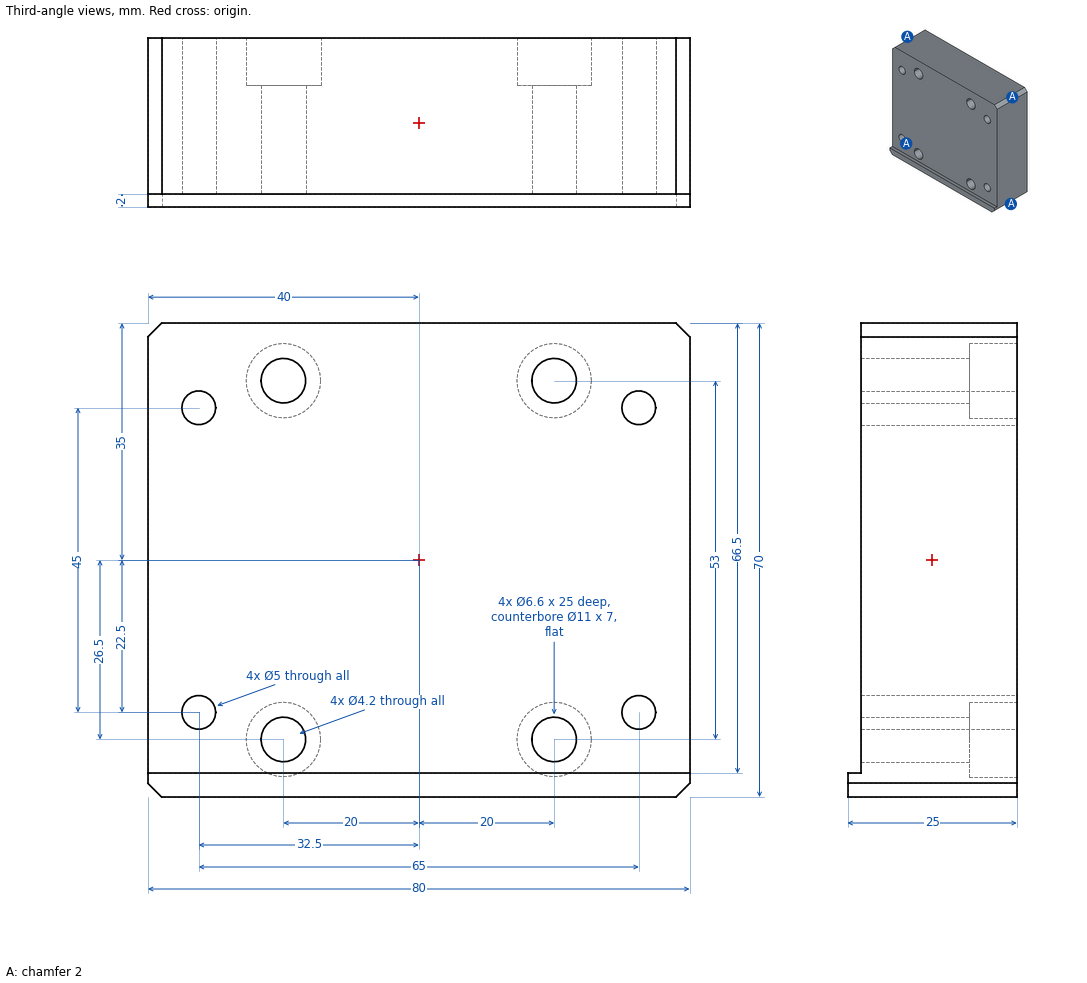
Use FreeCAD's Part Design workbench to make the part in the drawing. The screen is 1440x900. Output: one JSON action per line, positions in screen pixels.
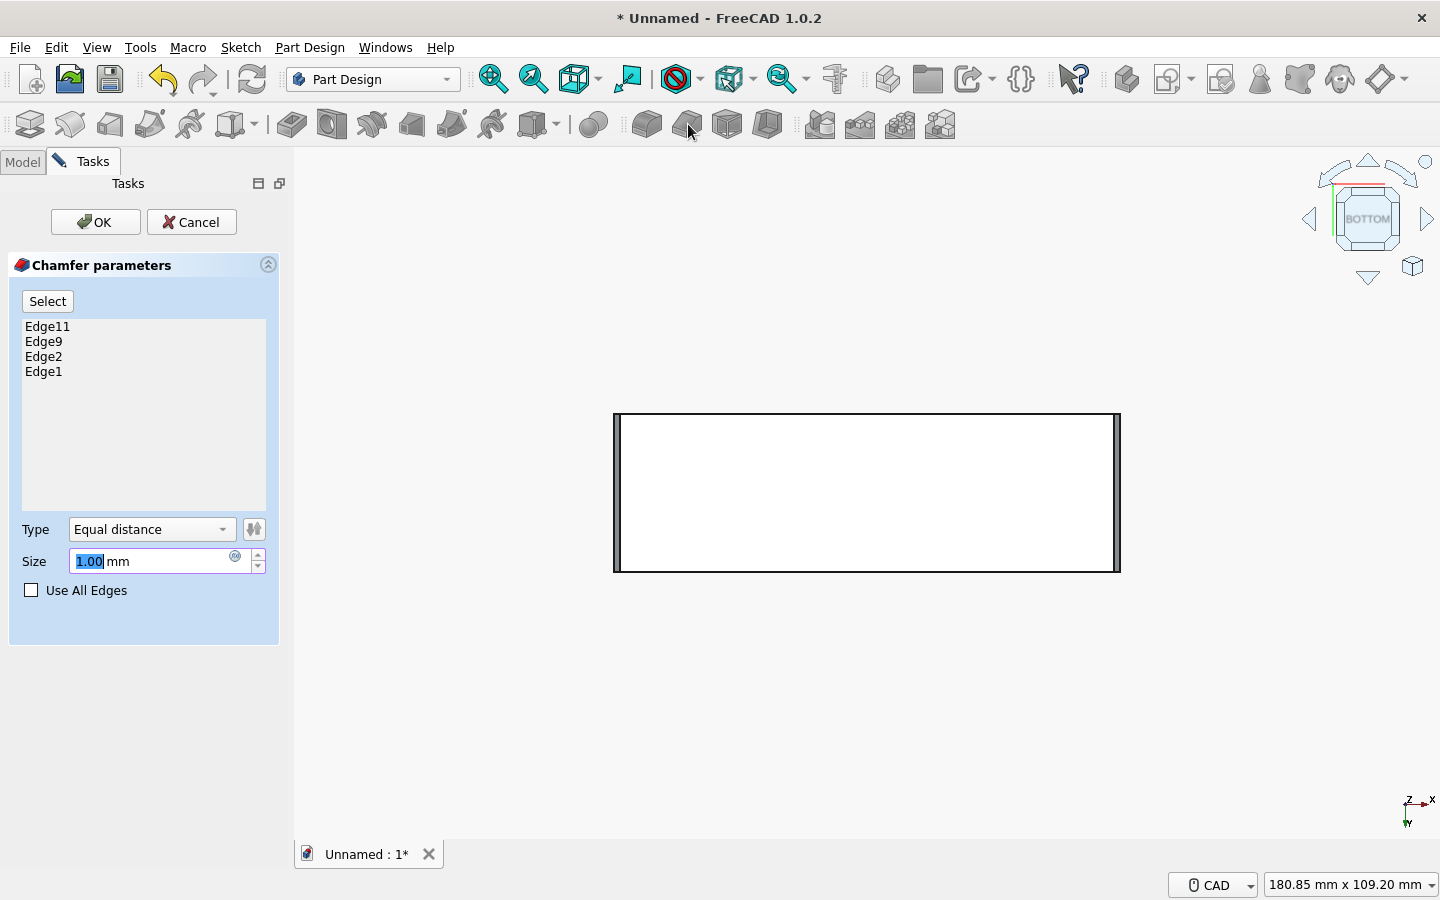
{"action": "type", "text": "2"}
{"action": "key", "text": "Tab"}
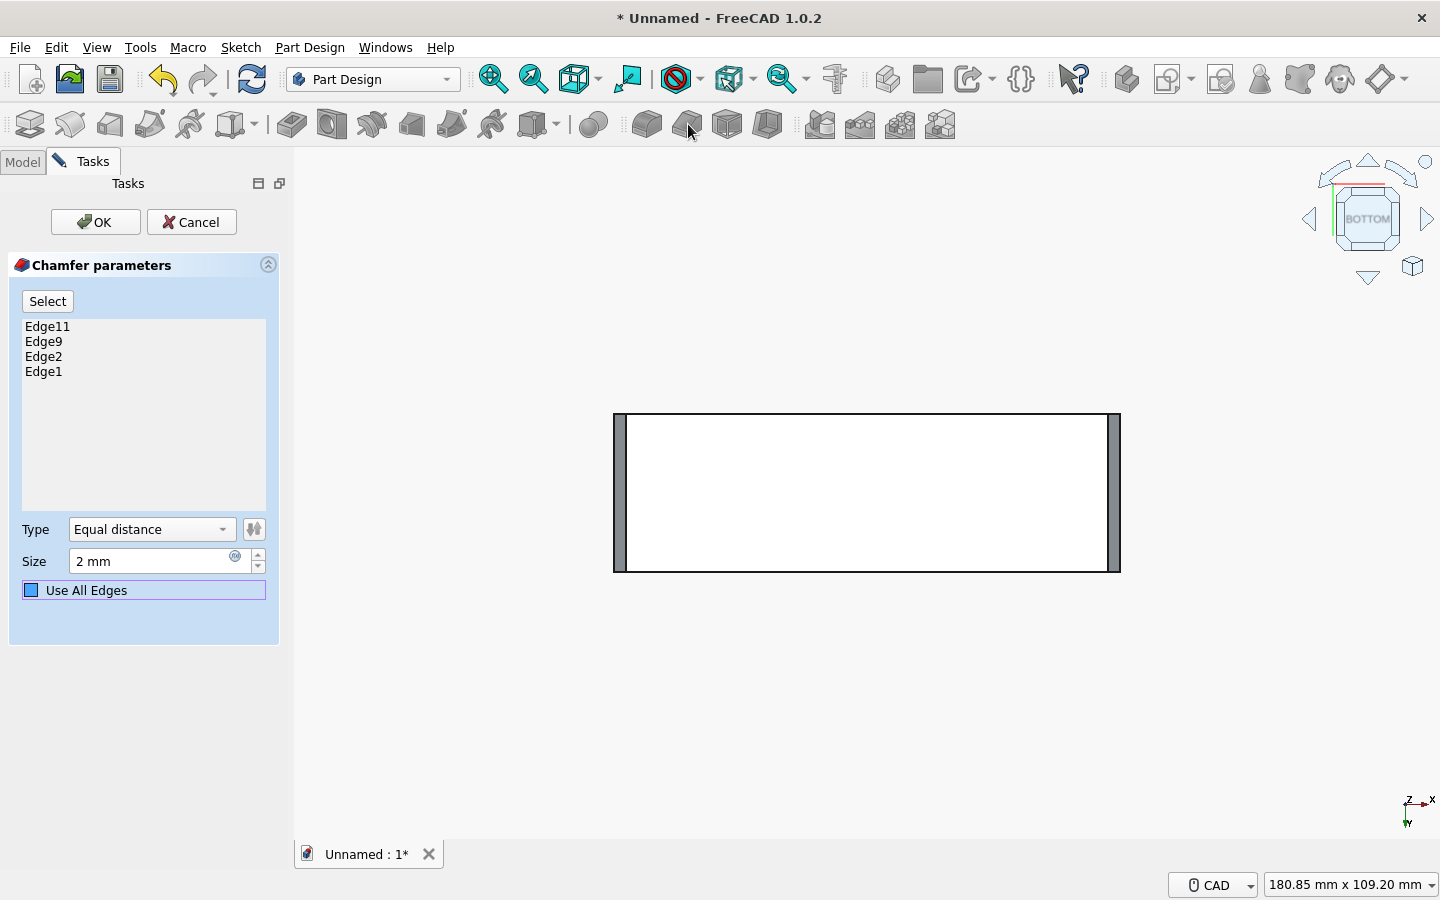
{"action": "left_click", "coordinate": [96, 222]}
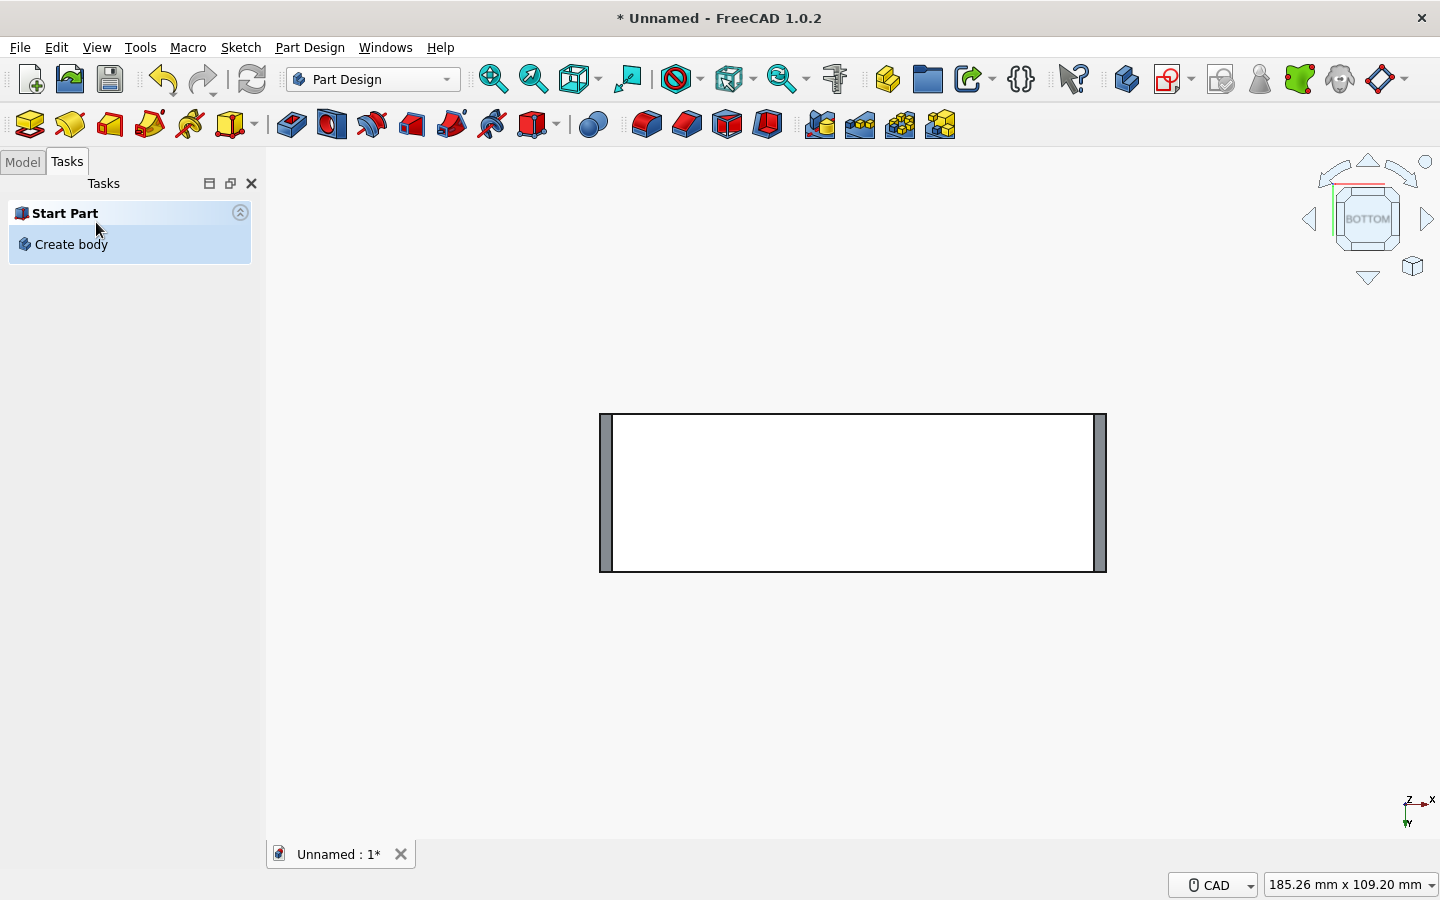
{"action": "left_click", "coordinate": [494, 80]}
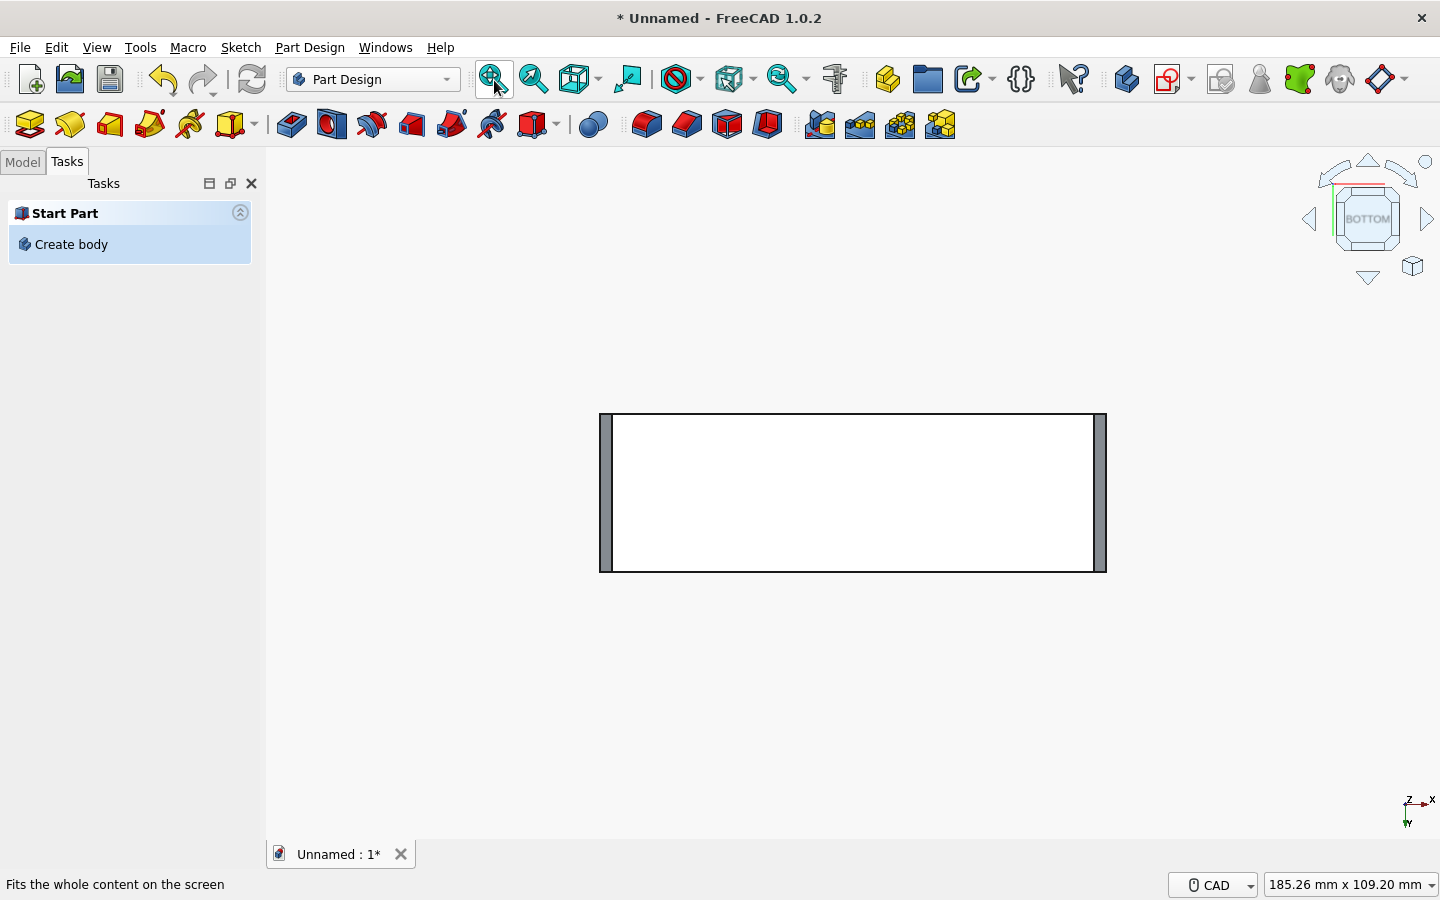
{"action": "key", "text": "4"}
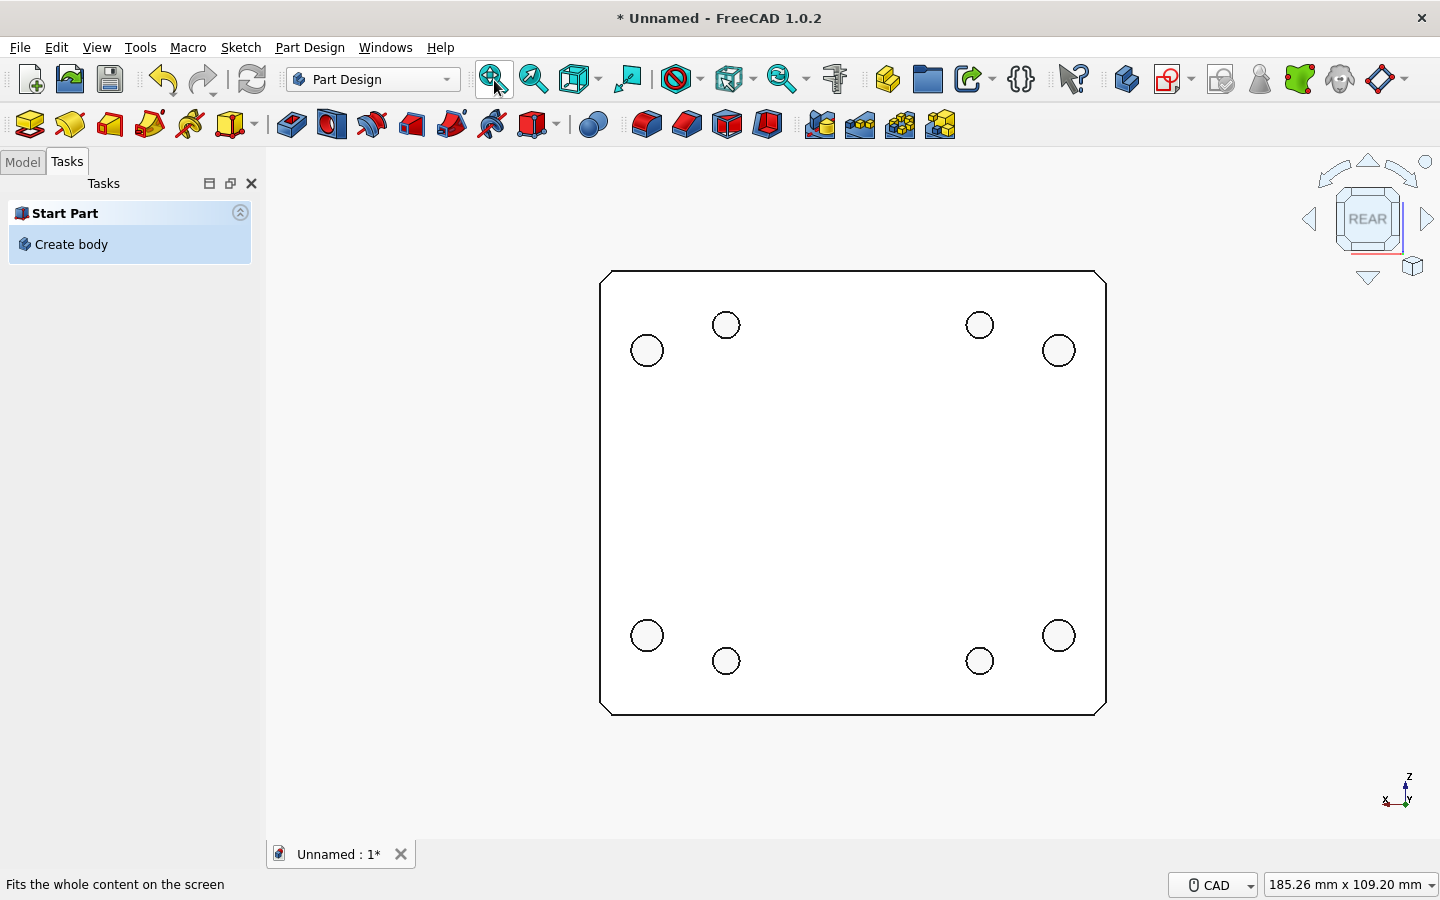
{"action": "left_click", "coordinate": [853, 492]}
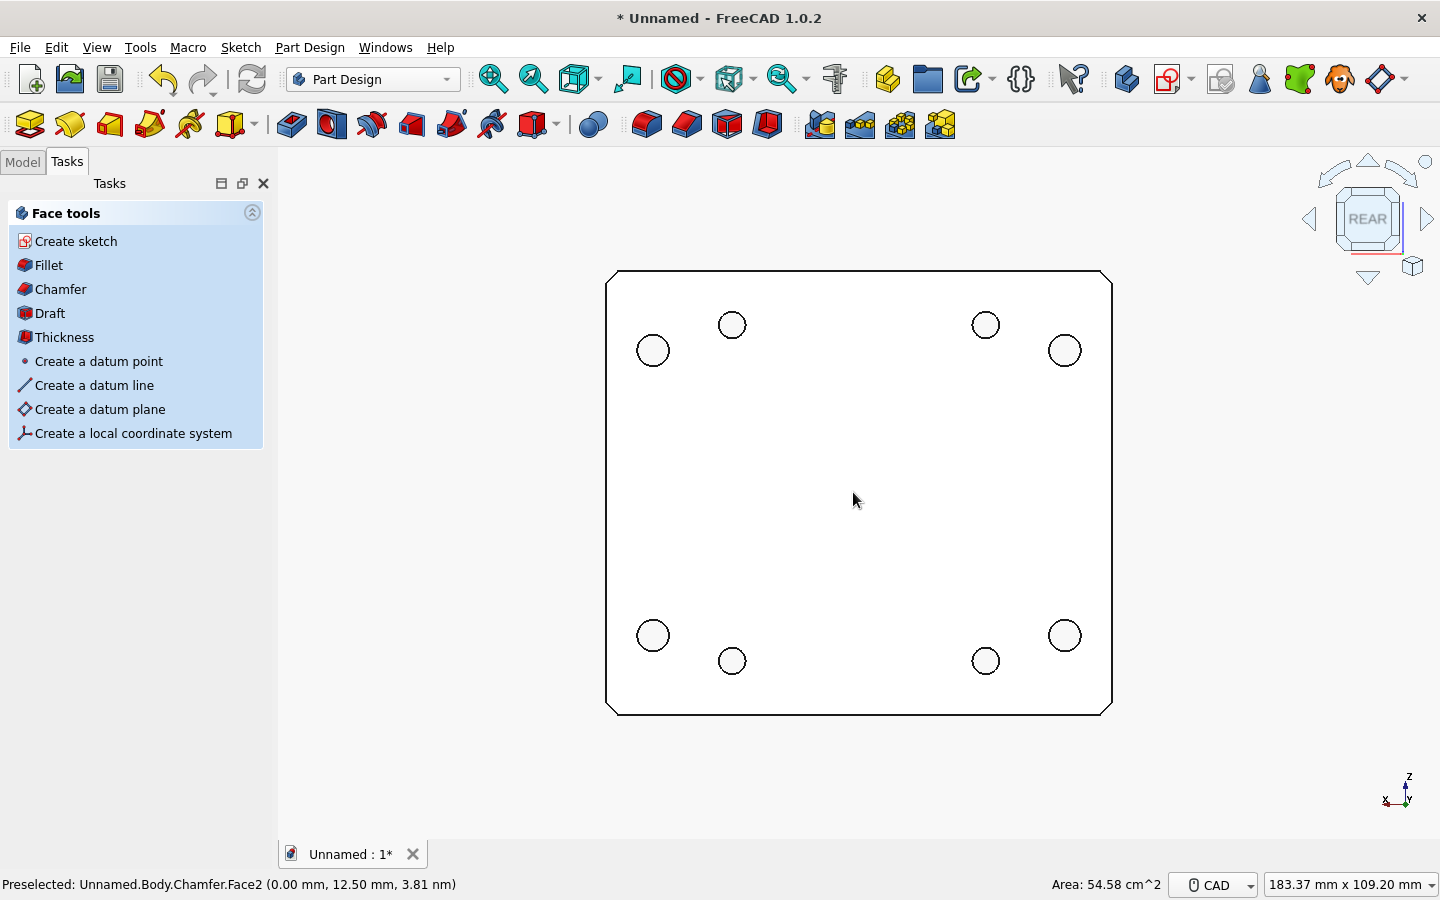
{"action": "left_click", "coordinate": [1168, 80]}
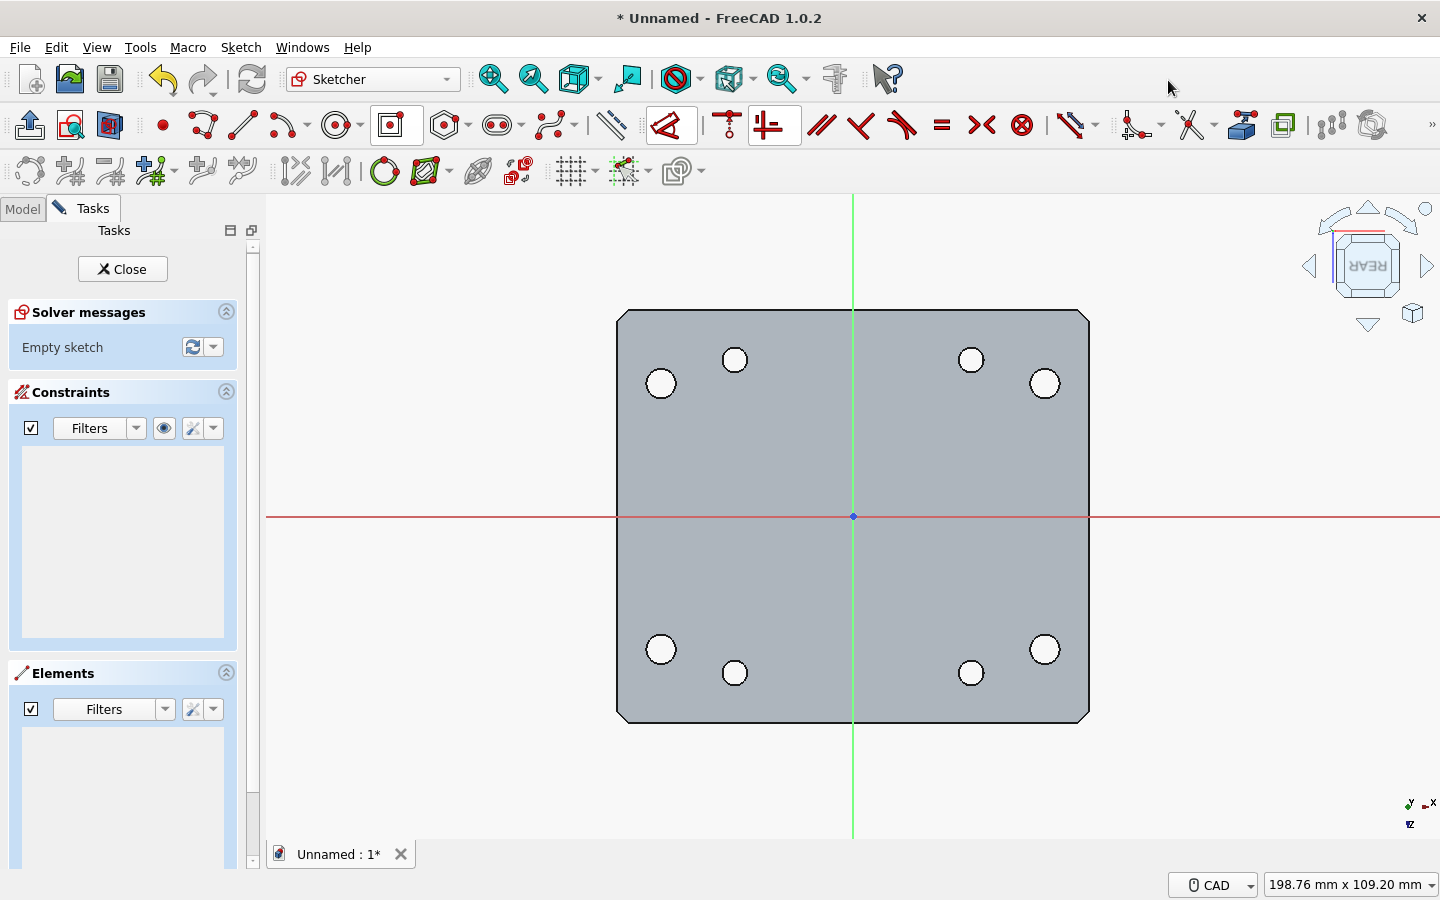
{"action": "left_click", "coordinate": [336, 126]}